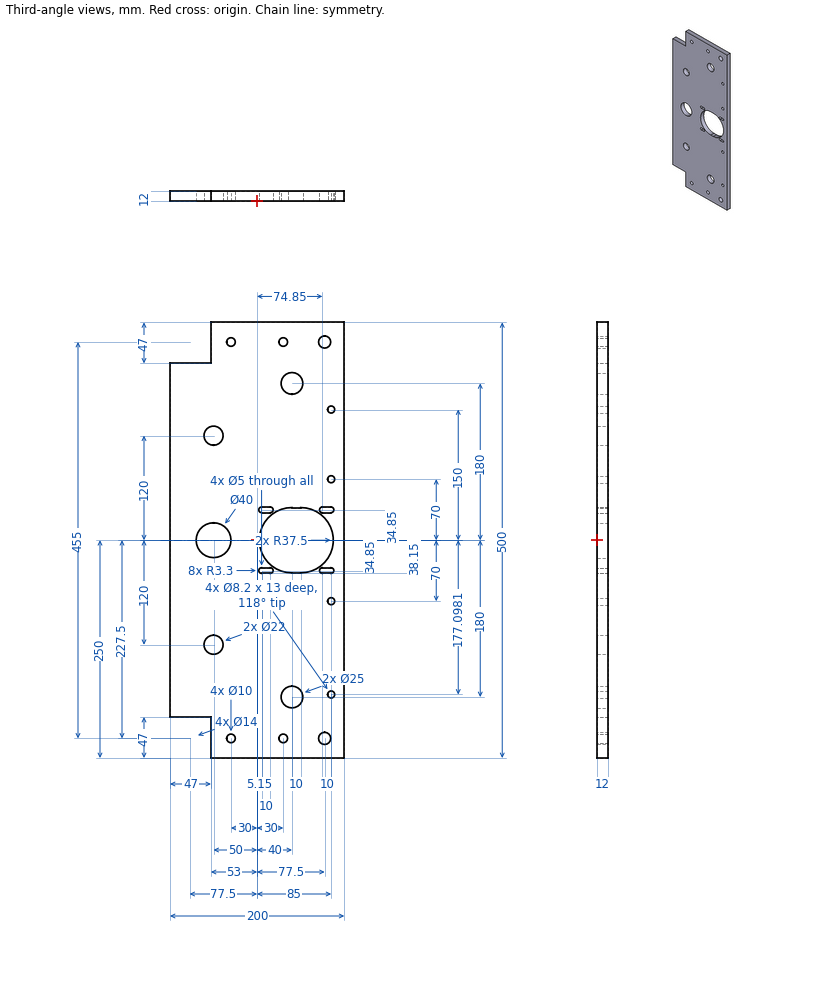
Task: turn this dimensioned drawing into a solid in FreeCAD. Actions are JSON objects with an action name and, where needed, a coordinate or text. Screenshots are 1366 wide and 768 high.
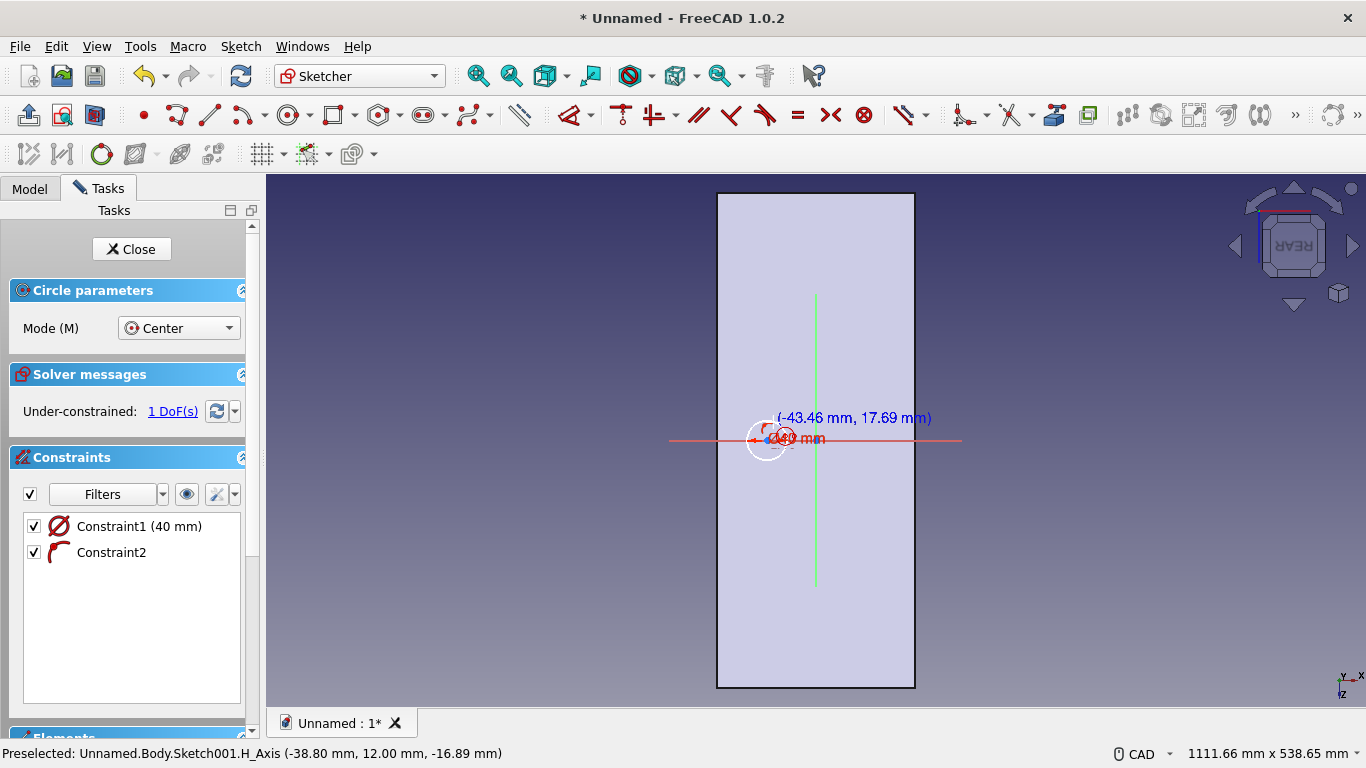
{"action": "scroll", "coordinate": [767, 322], "scroll_direction": "up", "scroll_amount": 4}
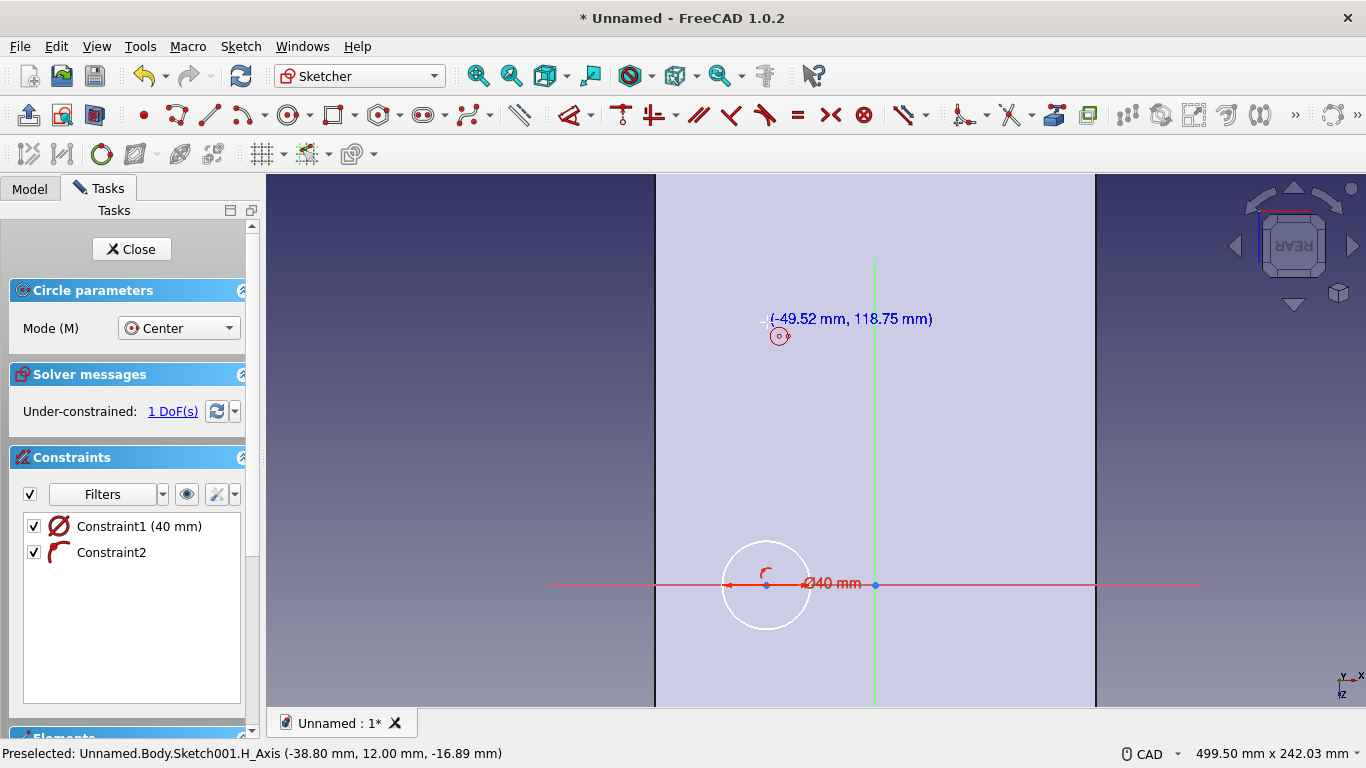
{"action": "left_click", "coordinate": [765, 321]}
{"action": "mouse_move", "coordinate": [783, 304]}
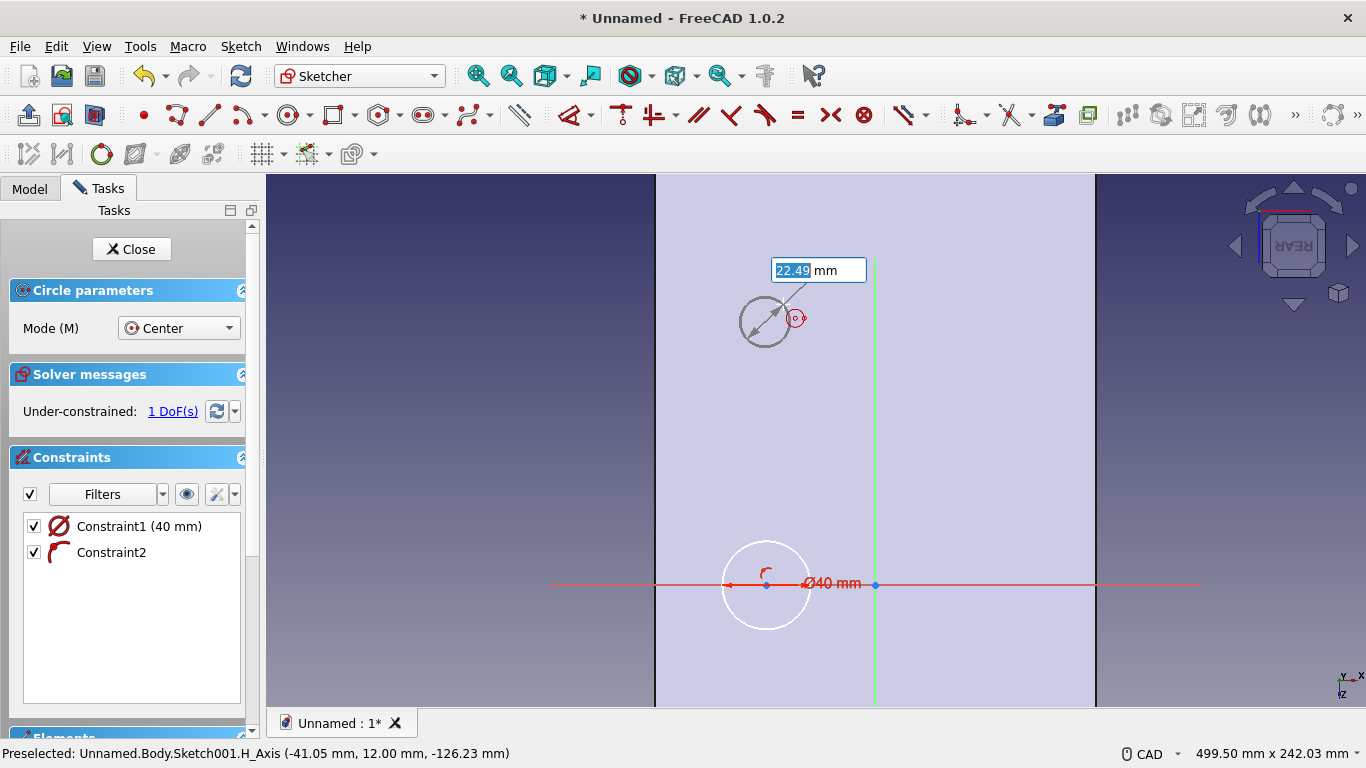
{"action": "type", "text": "22"}
{"action": "key", "text": "Return"}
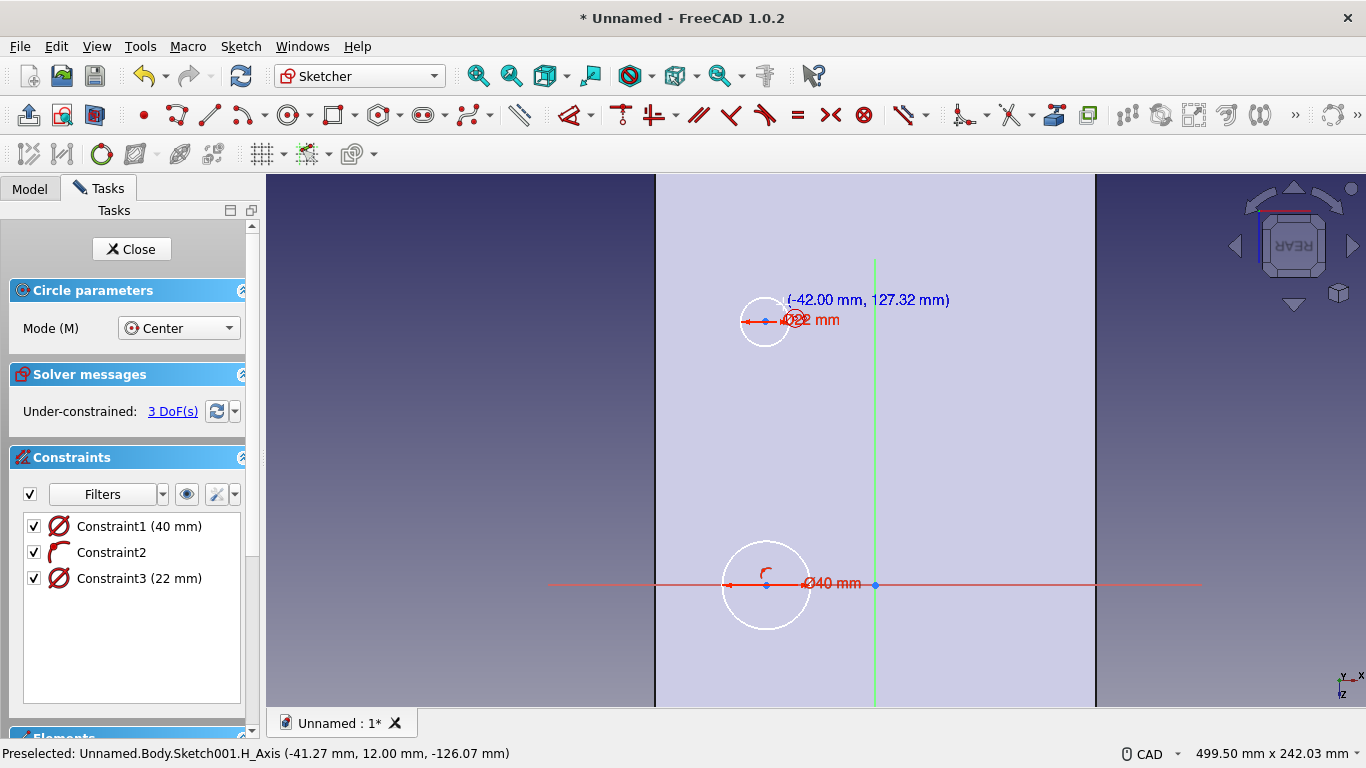
{"action": "scroll", "coordinate": [686, 264], "scroll_direction": "down", "scroll_amount": 3}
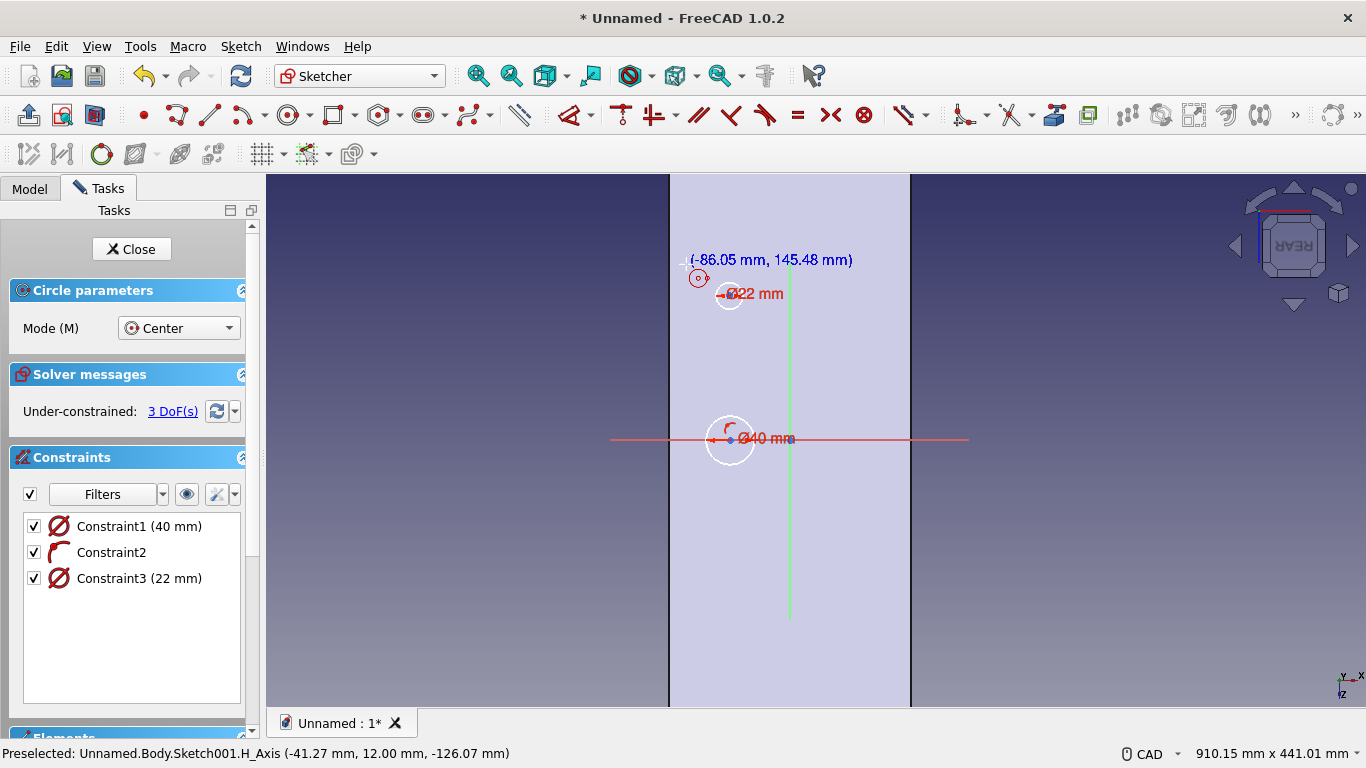
{"action": "scroll", "coordinate": [730, 585], "scroll_direction": "up", "scroll_amount": 3}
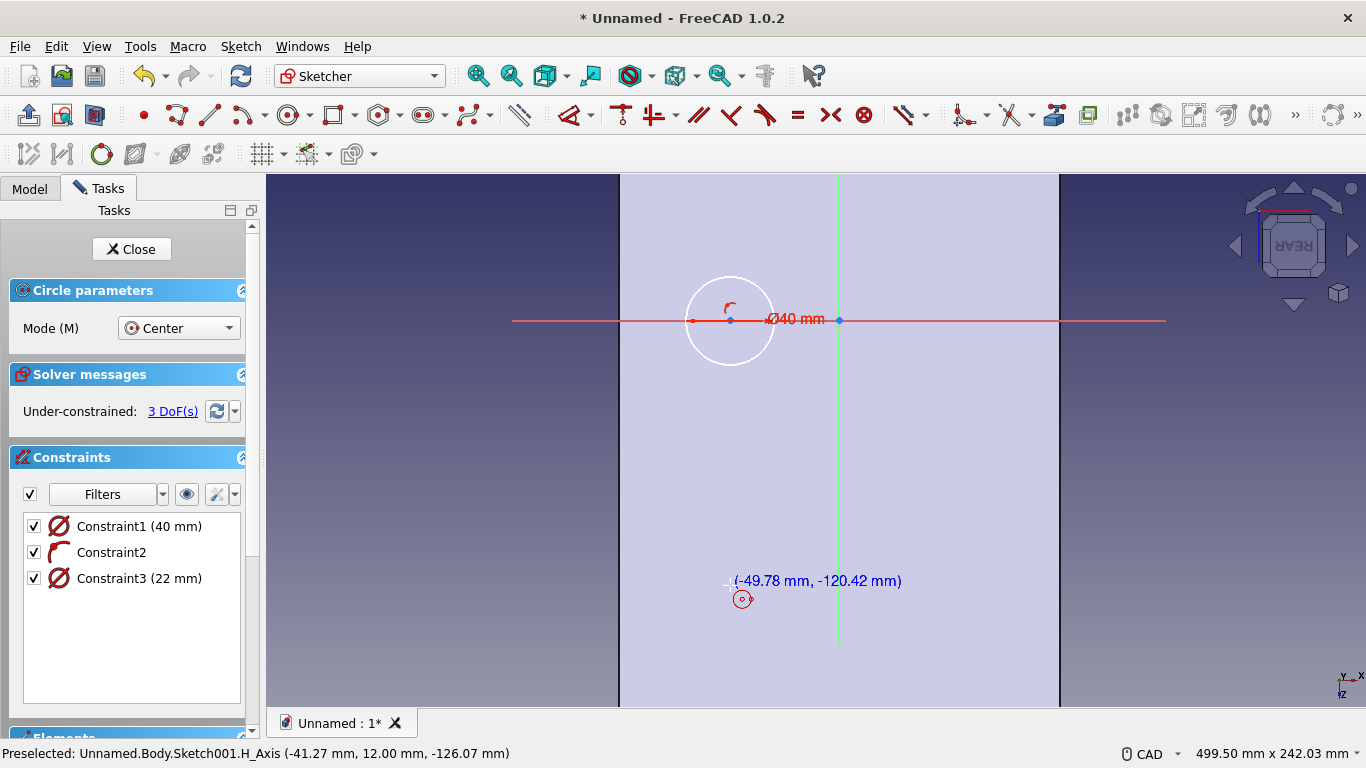
{"action": "left_click", "coordinate": [729, 585]}
{"action": "mouse_move", "coordinate": [746, 568]}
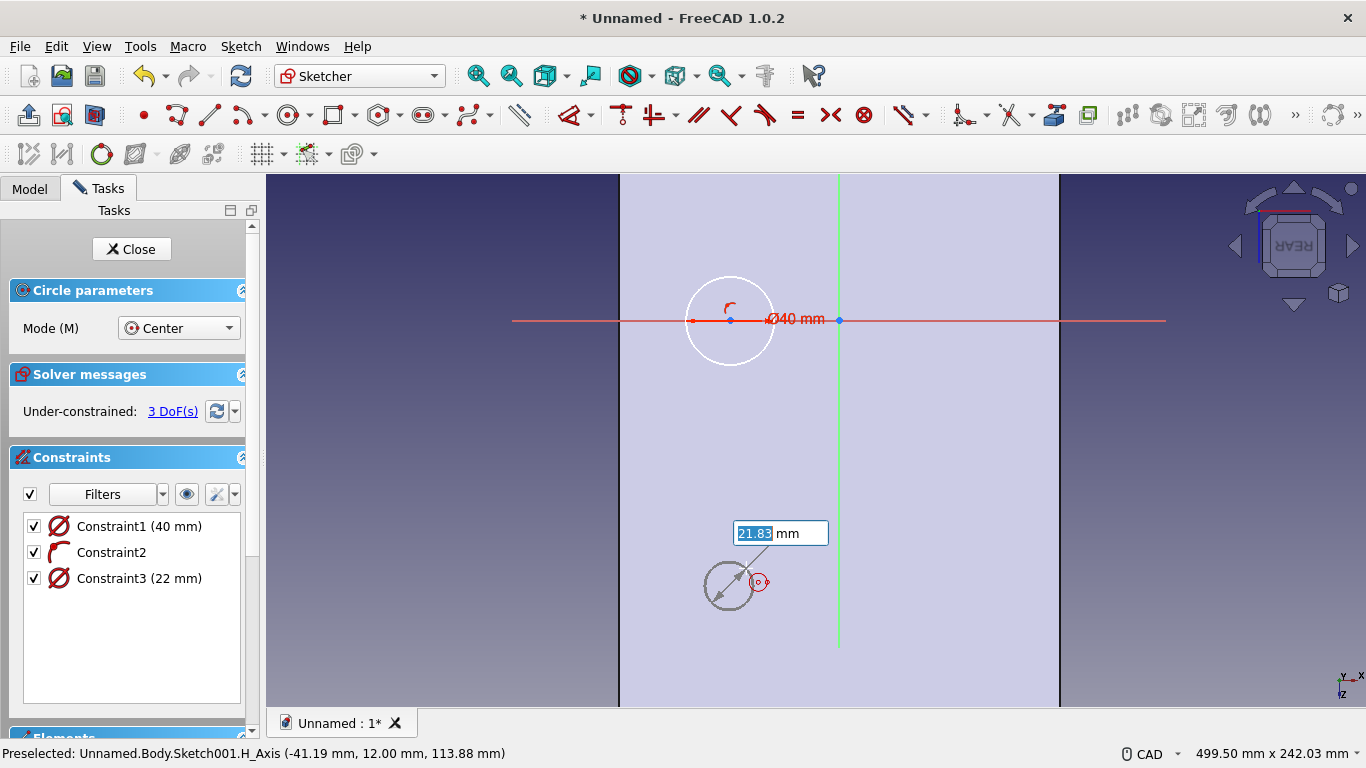
{"action": "type", "text": "22"}
{"action": "key", "text": "Return"}
{"action": "key", "text": "Escape"}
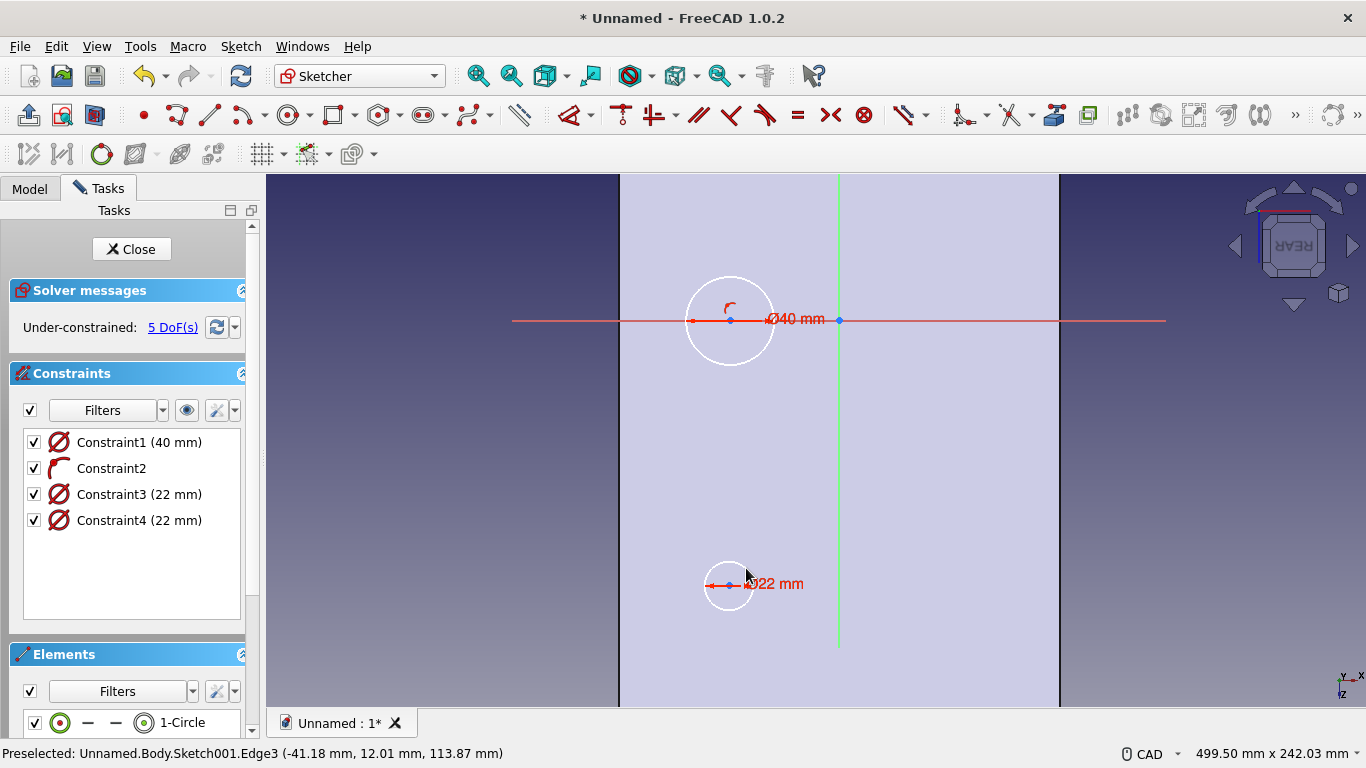
{"action": "left_click", "coordinate": [730, 321]}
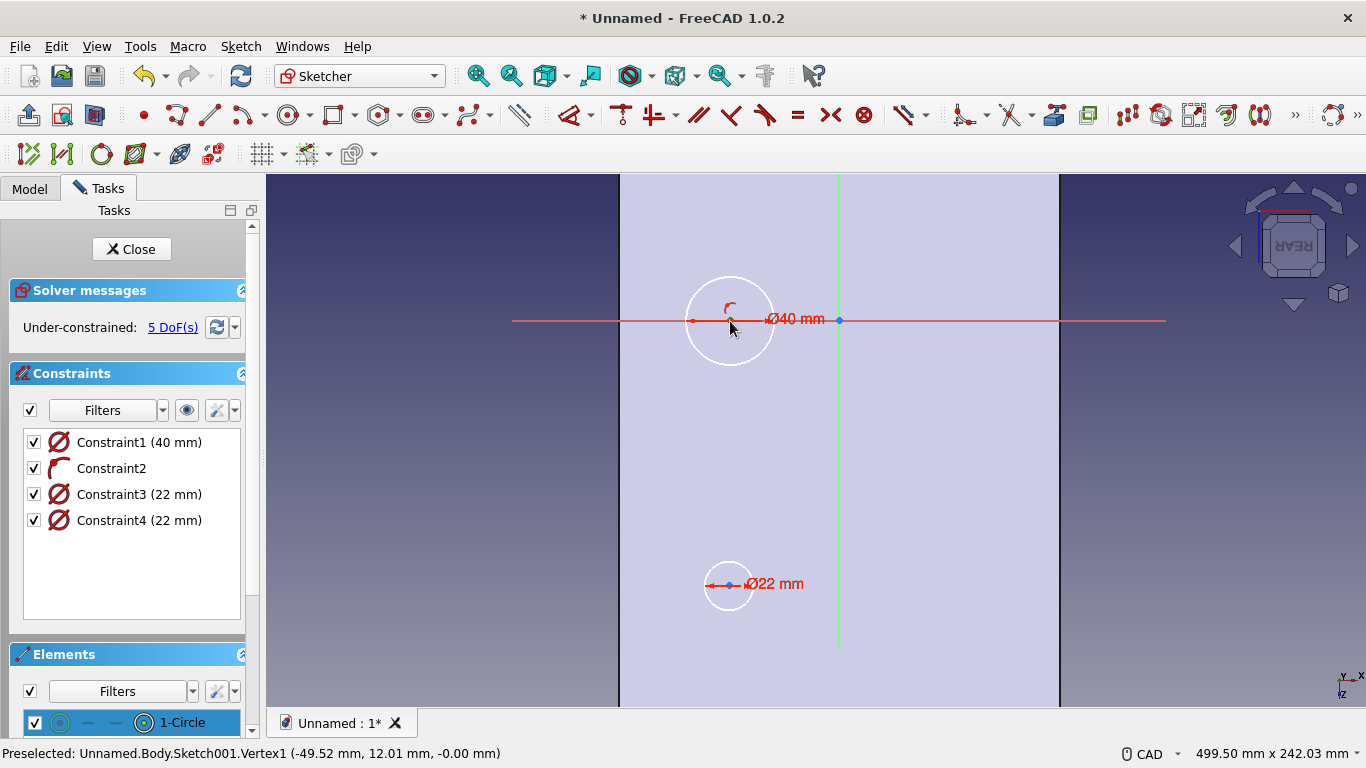
{"action": "scroll", "coordinate": [730, 586], "scroll_direction": "down", "scroll_amount": 3}